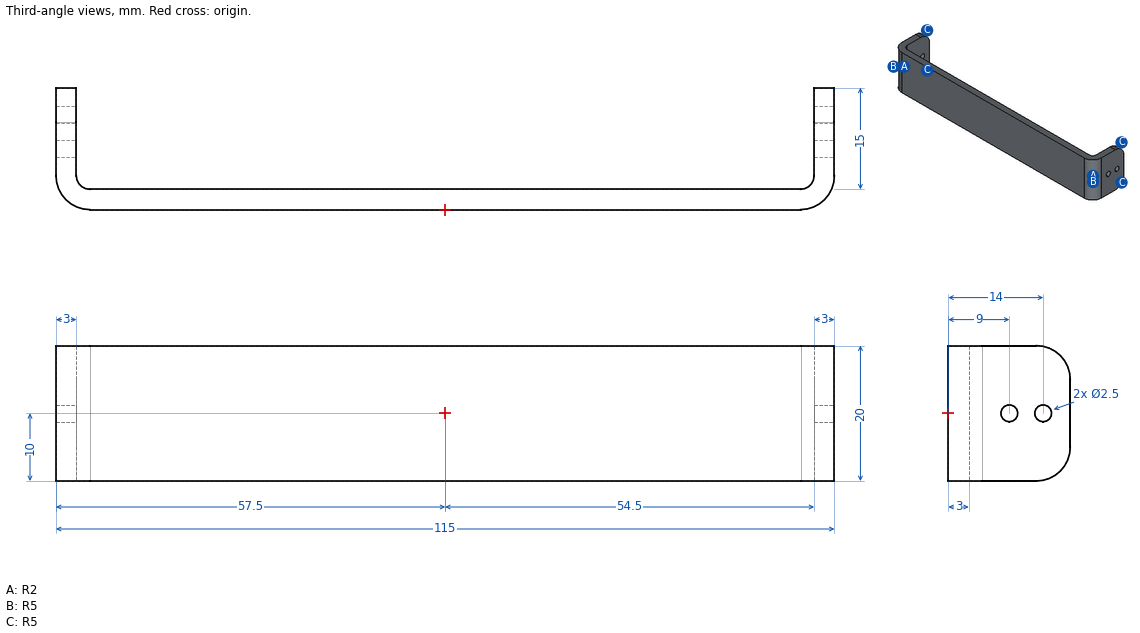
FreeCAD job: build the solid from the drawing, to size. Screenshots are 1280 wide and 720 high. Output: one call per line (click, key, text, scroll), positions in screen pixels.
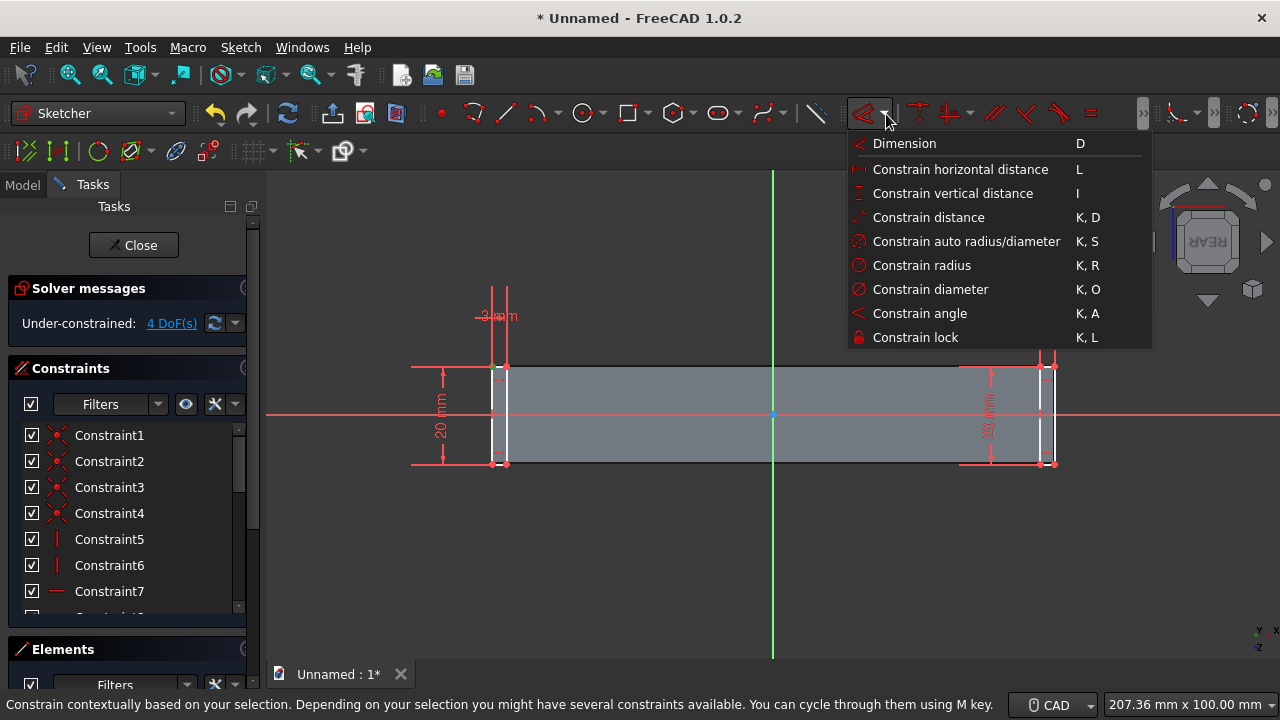
click(1000, 193)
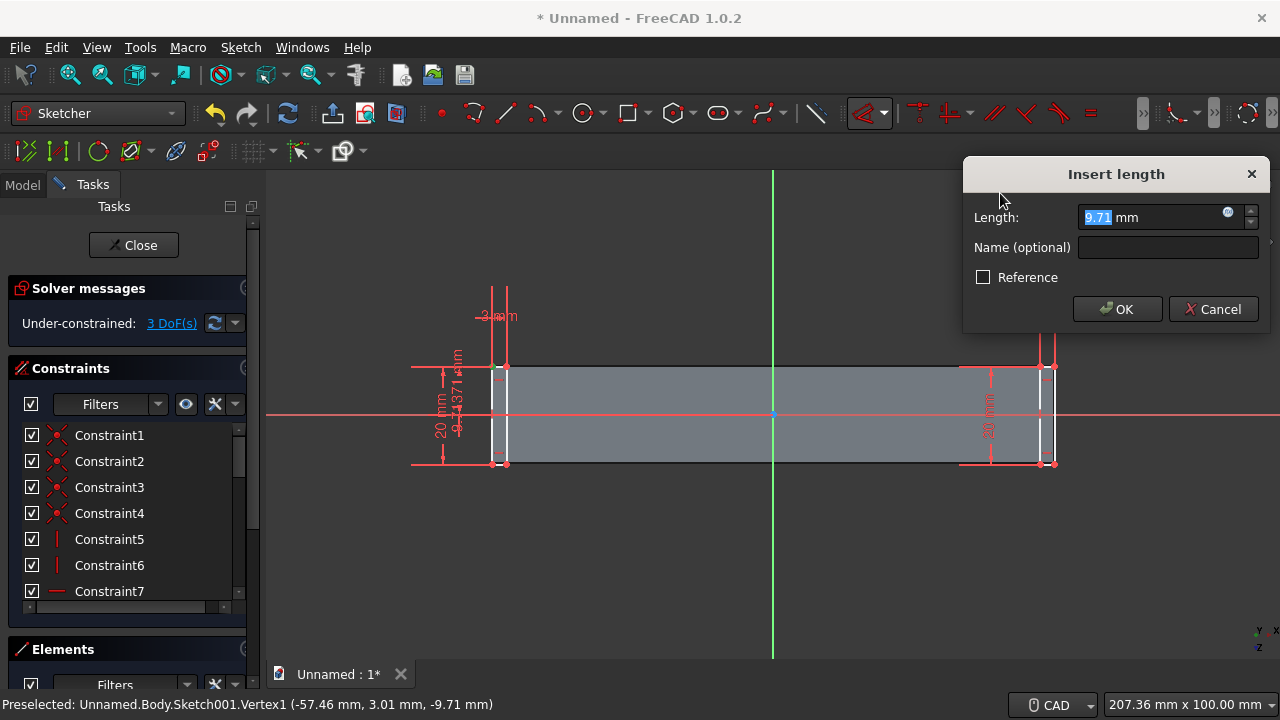
text(10)
key(Return)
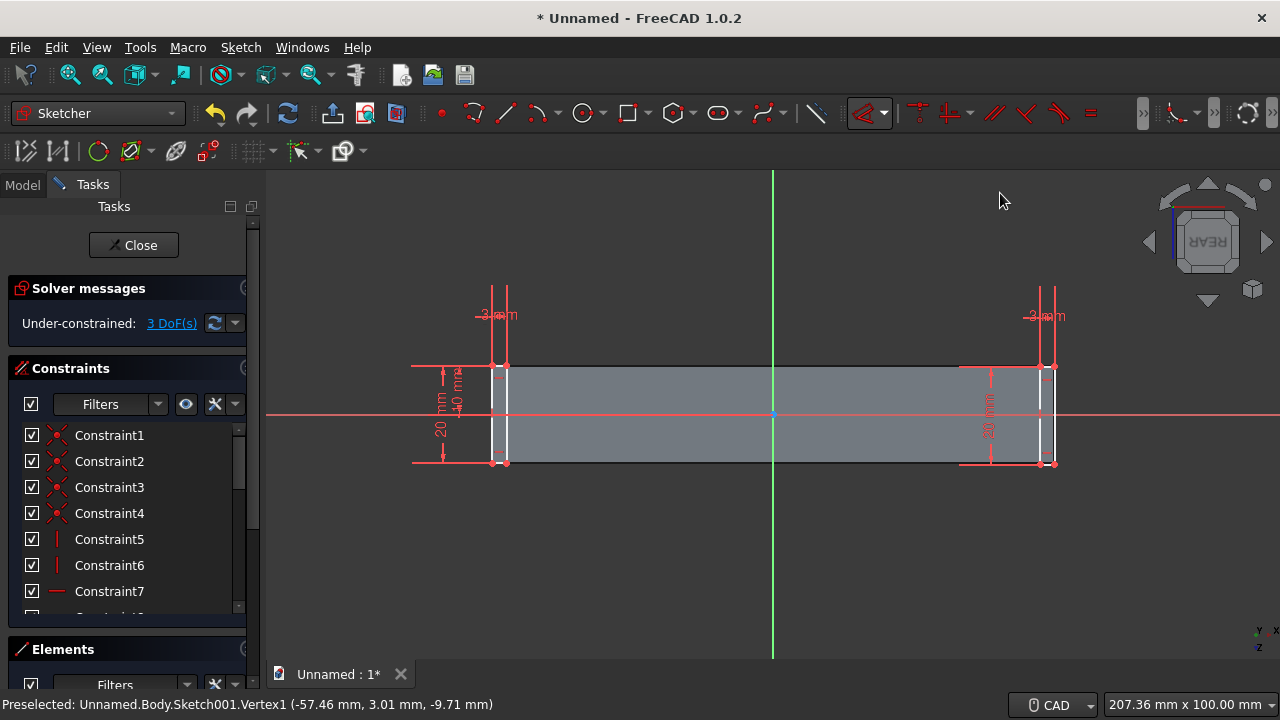
click(1040, 367)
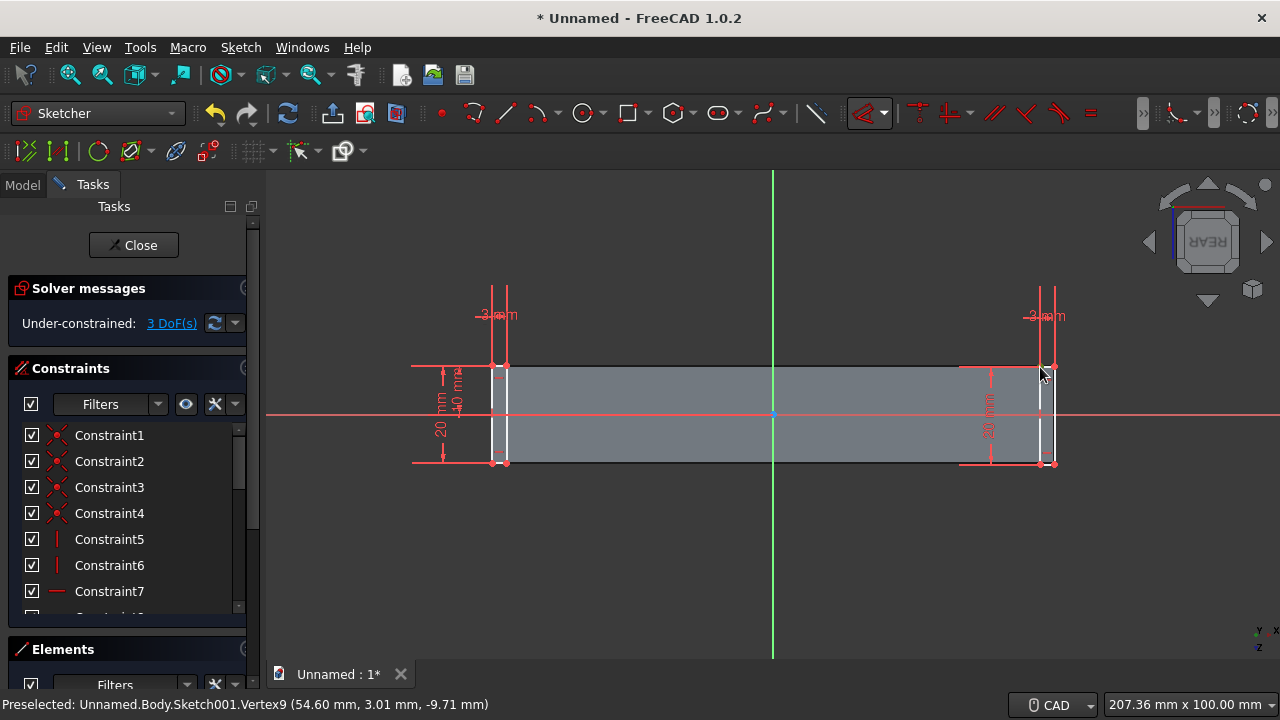
key(i)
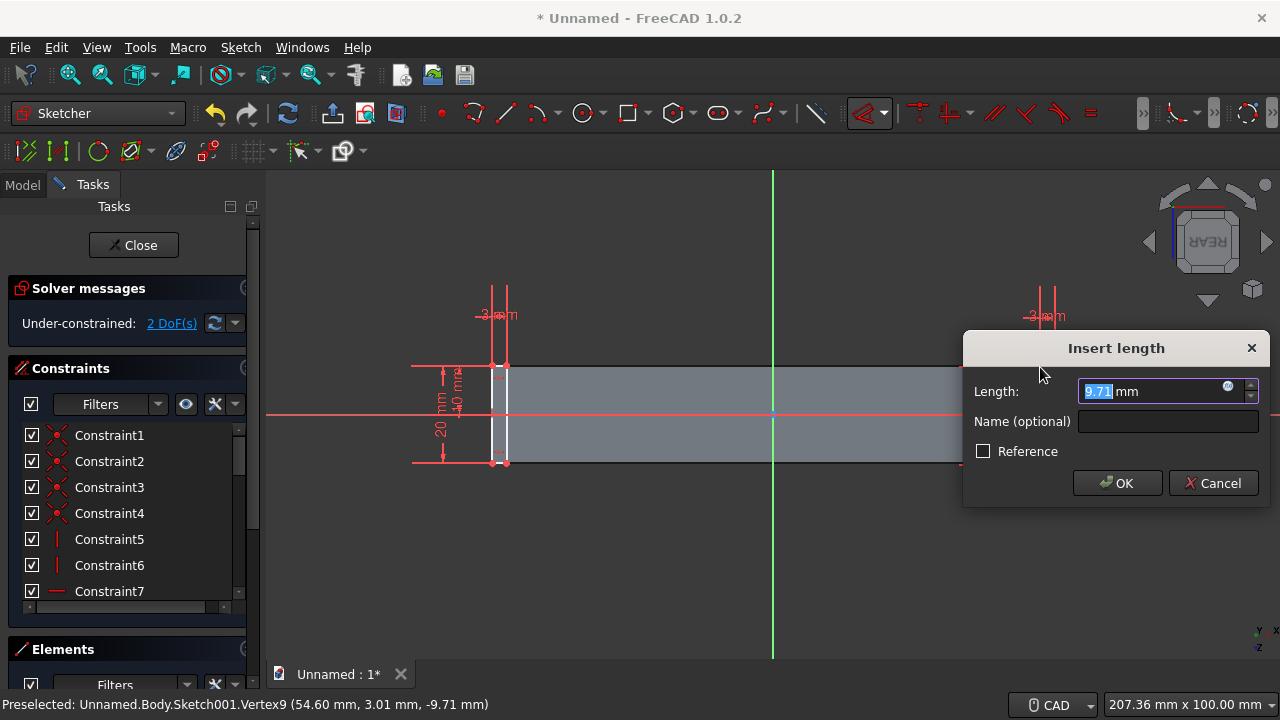
text(10)
key(Return)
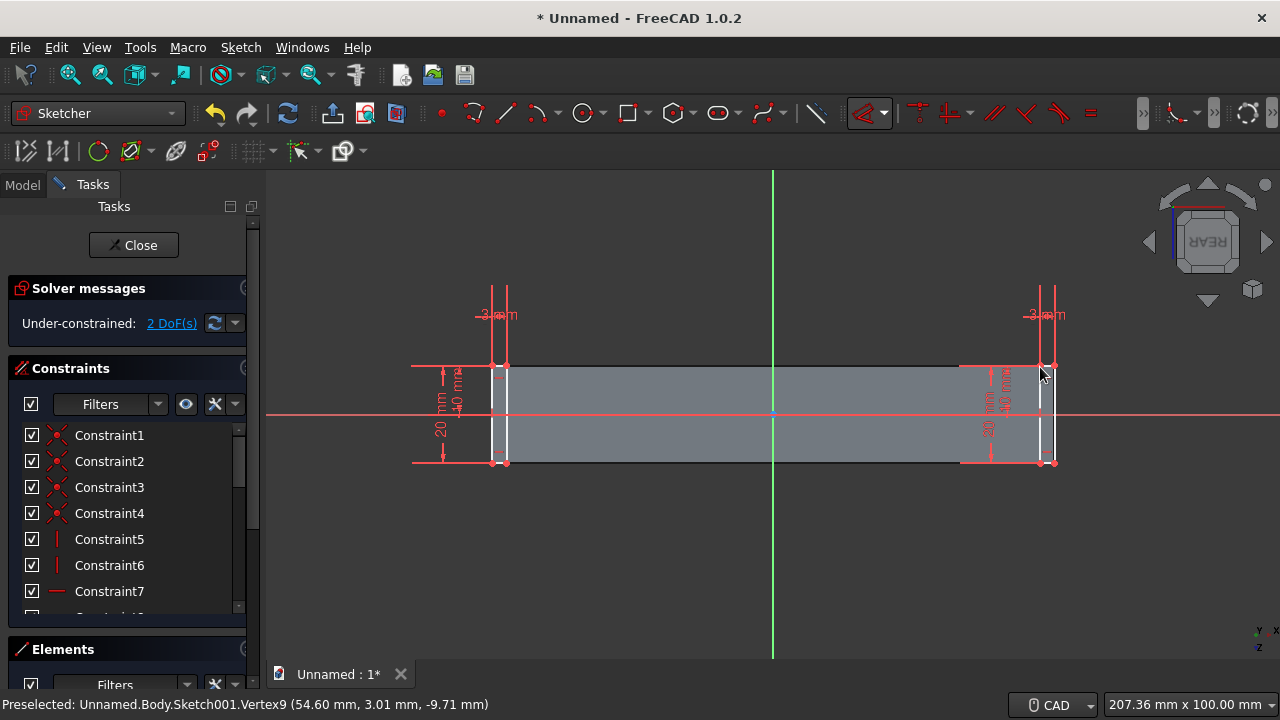
click(492, 366)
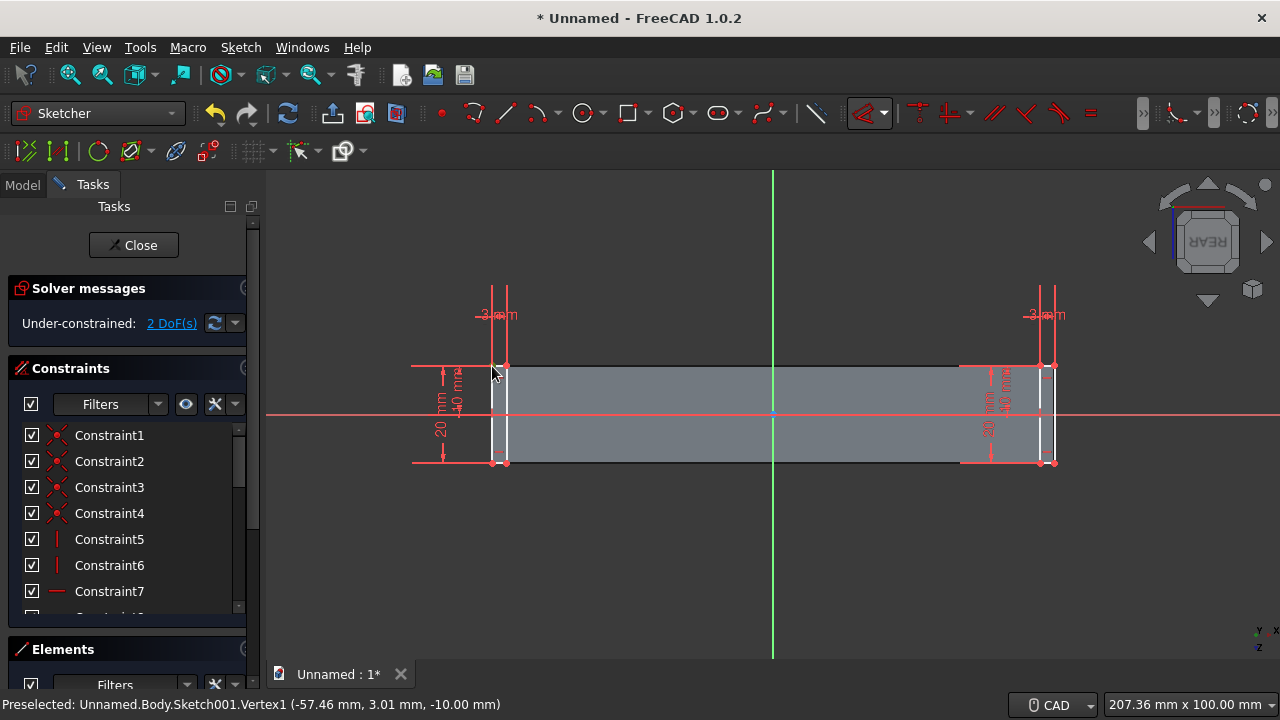
click(886, 114)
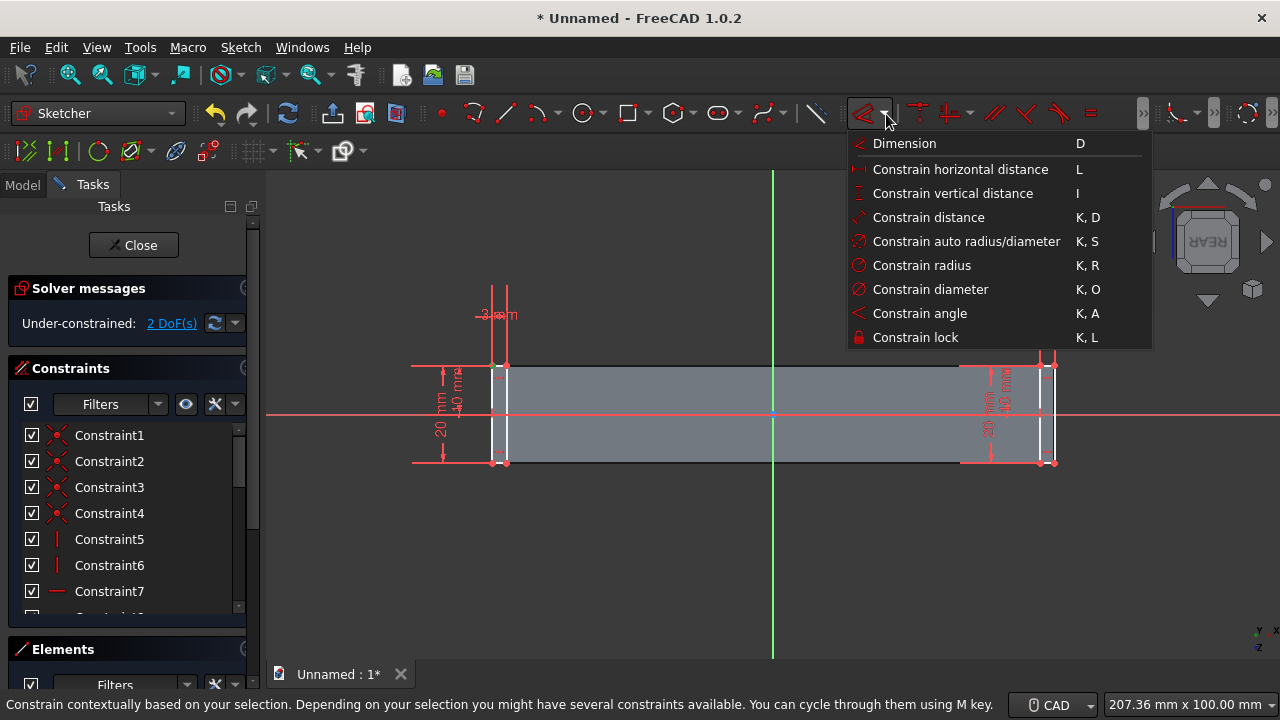
click(1000, 169)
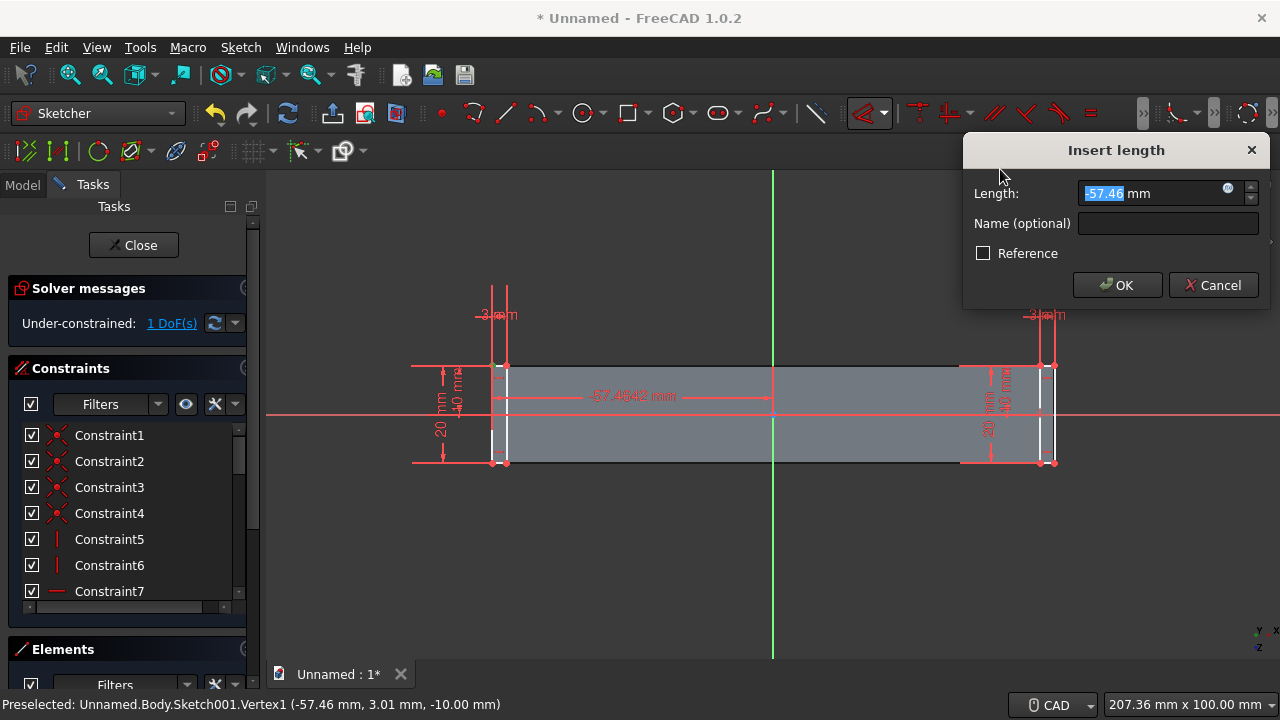
text(-57.5)
key(Return)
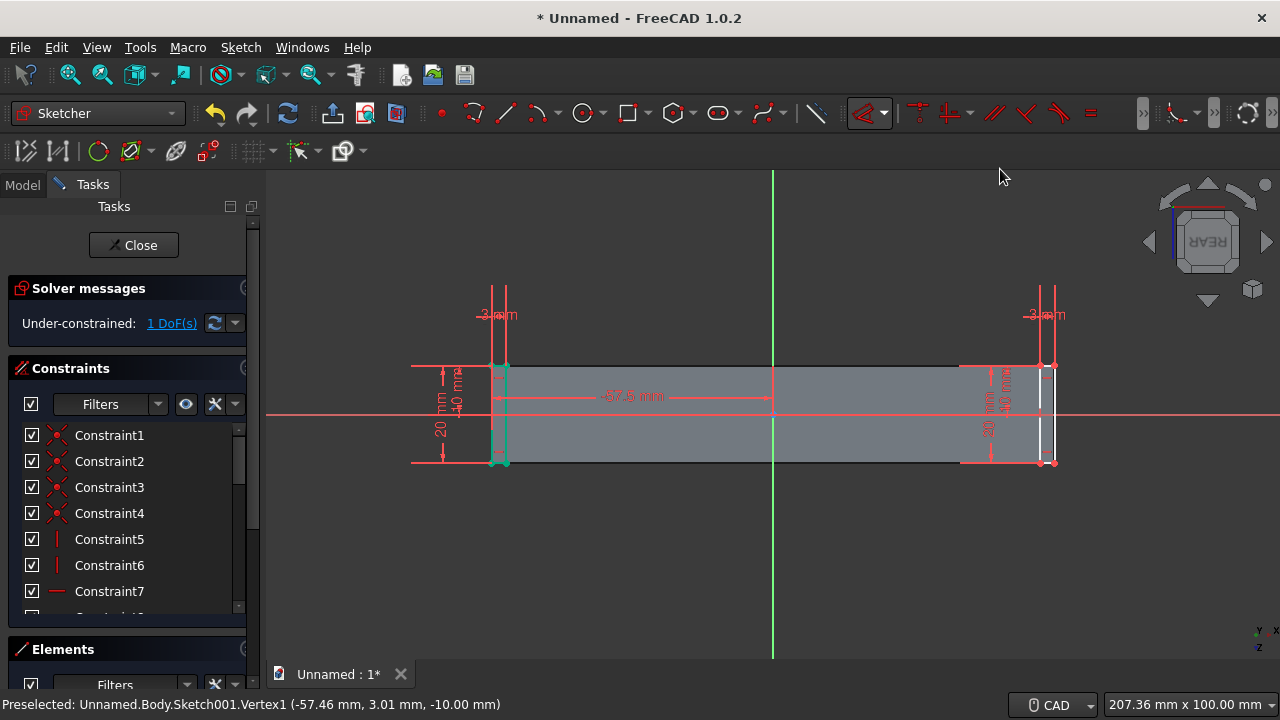
click(1040, 366)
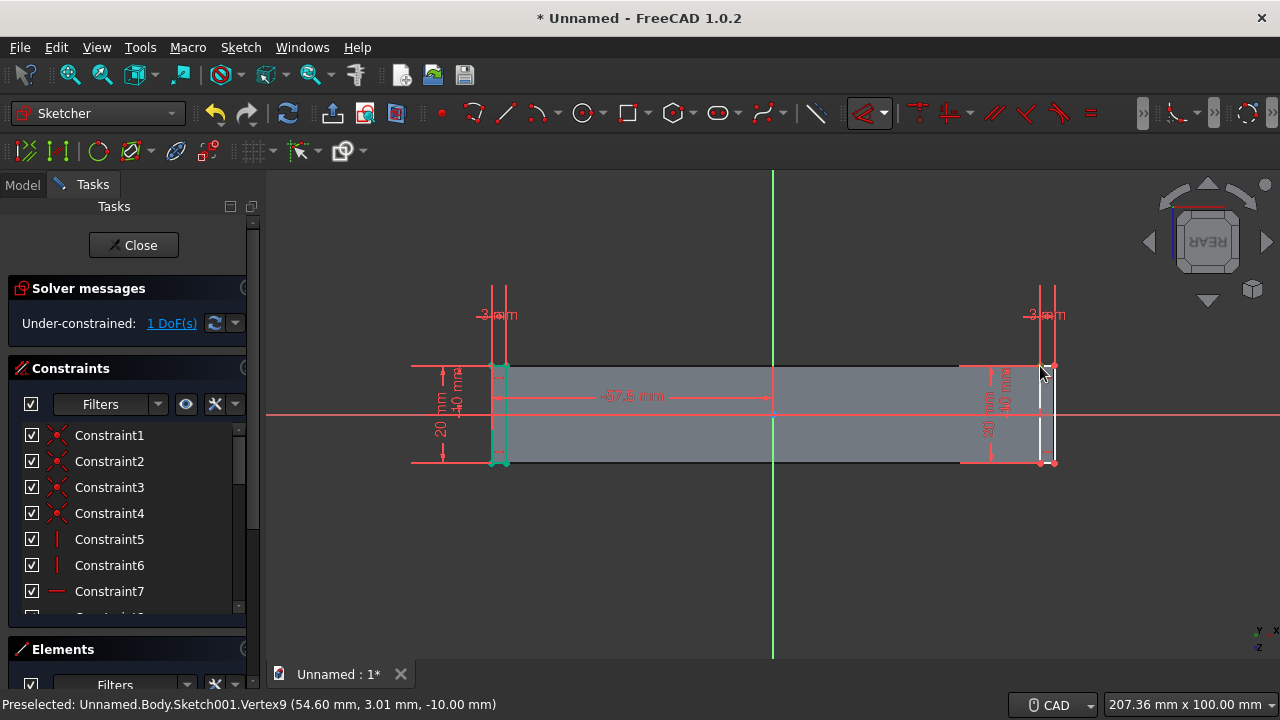
click(886, 114)